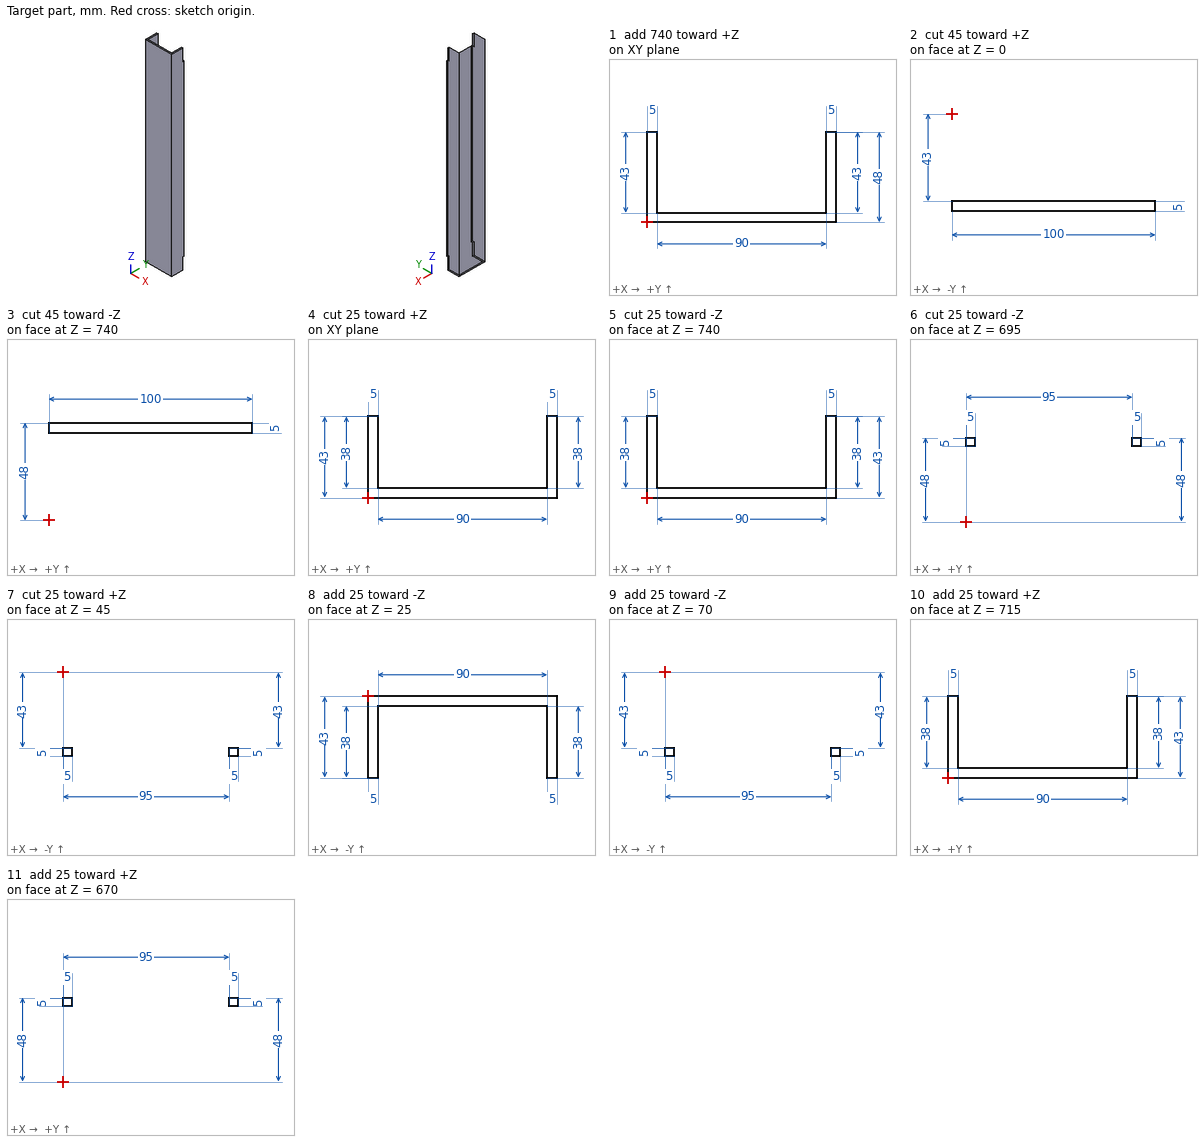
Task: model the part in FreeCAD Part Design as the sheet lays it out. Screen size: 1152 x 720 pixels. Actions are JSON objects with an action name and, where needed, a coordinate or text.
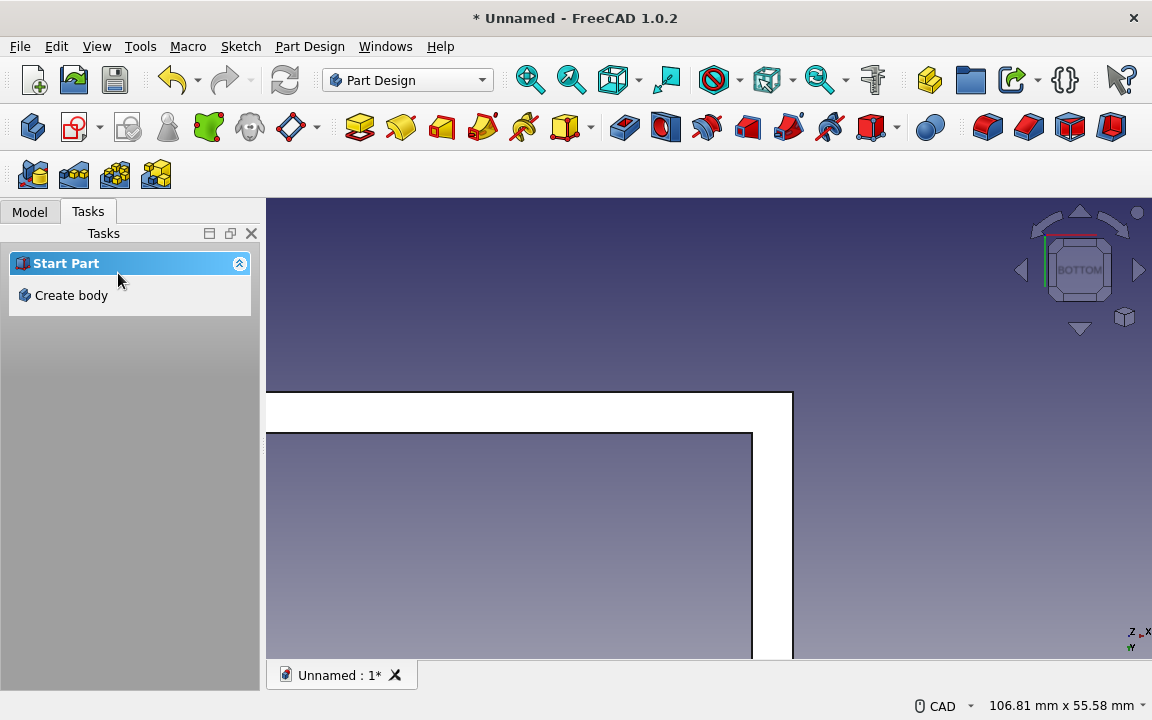
{"action": "left_click", "coordinate": [531, 80]}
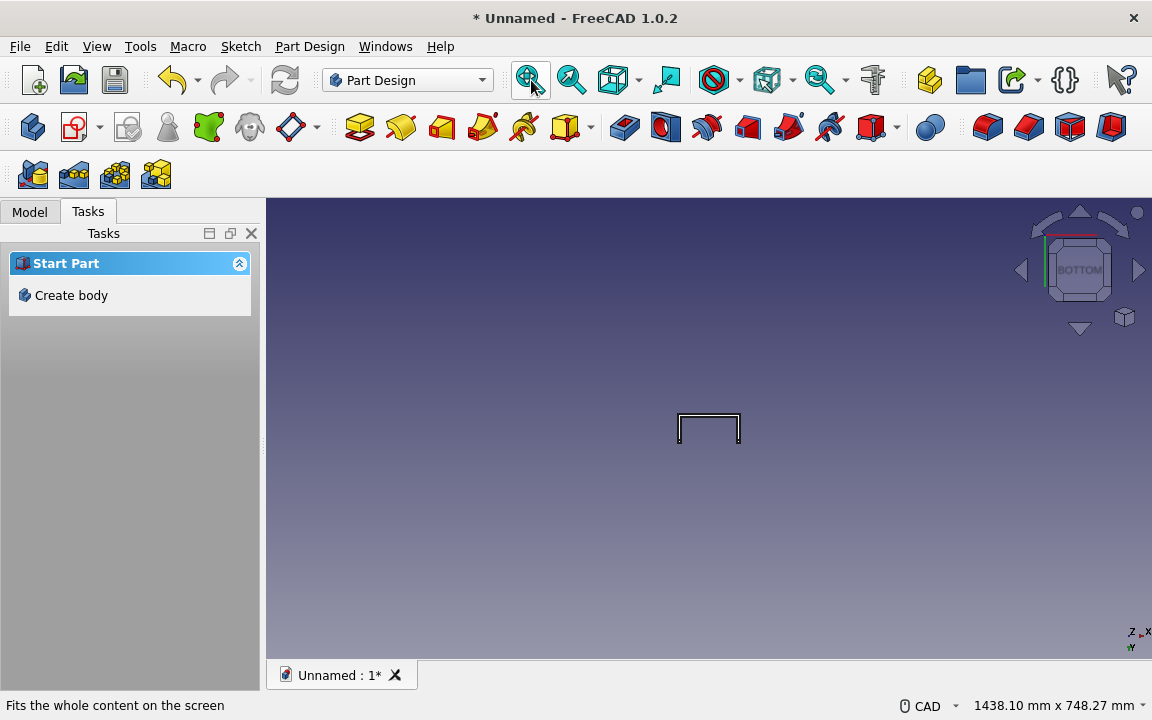
{"action": "key", "text": "0"}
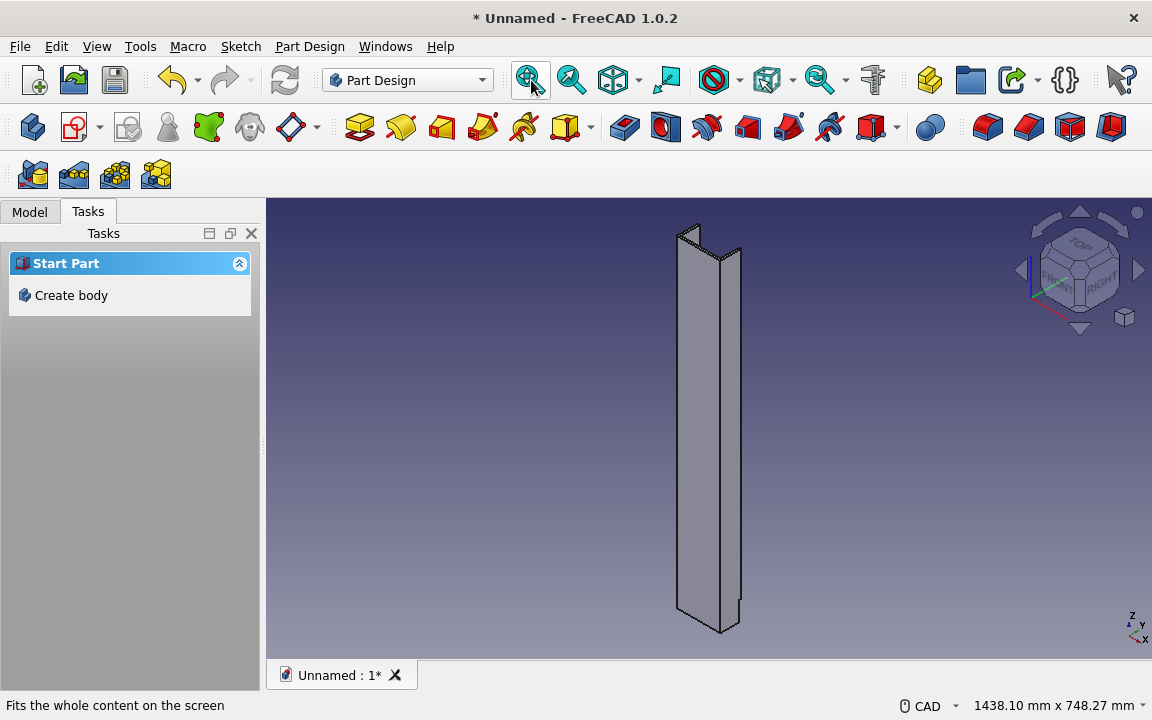
{"action": "scroll", "coordinate": [719, 257], "scroll_direction": "up", "scroll_amount": 13}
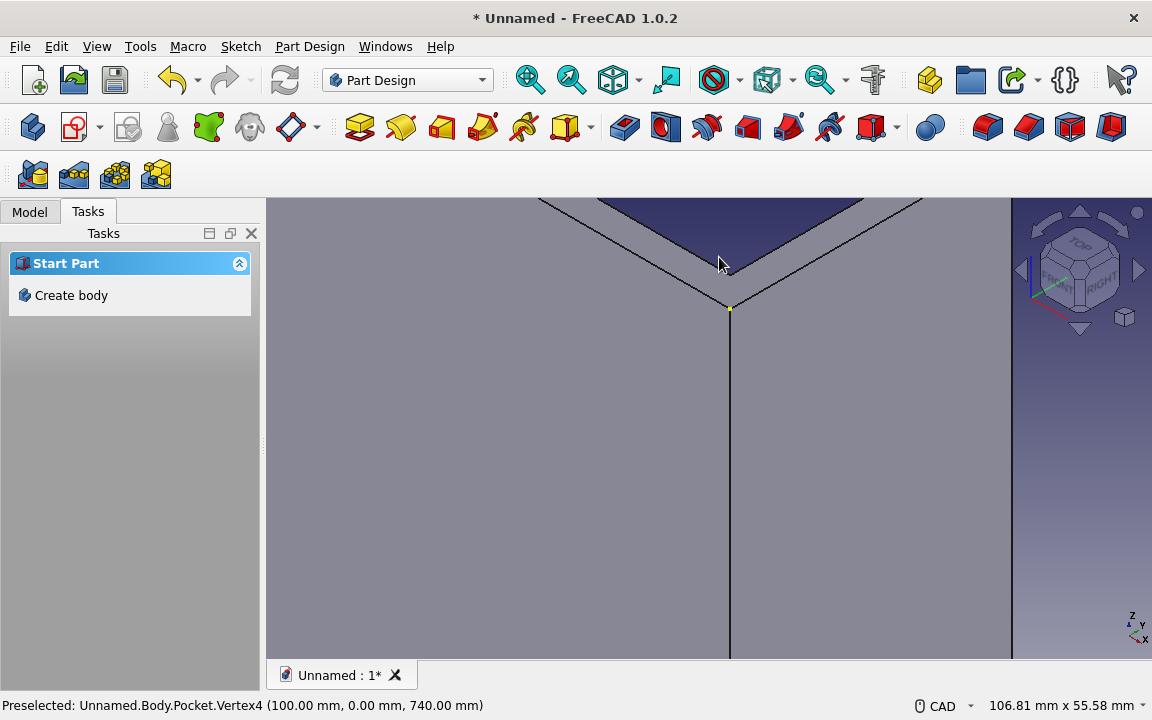
{"action": "left_click", "coordinate": [709, 272]}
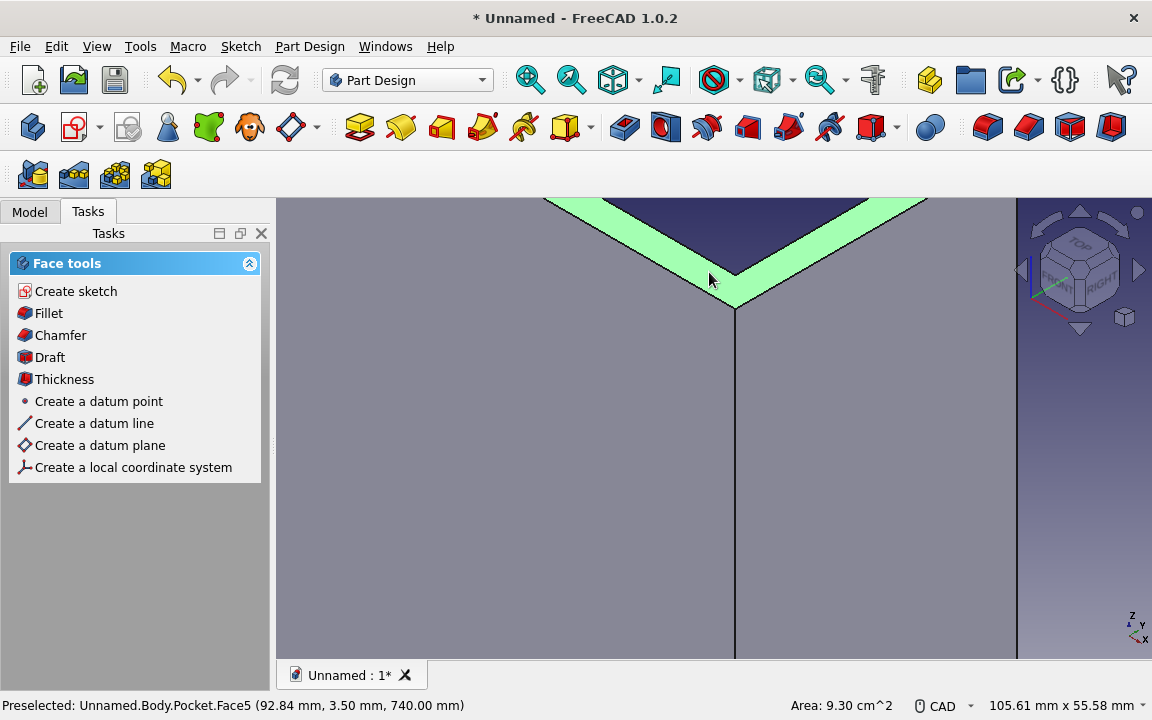
{"action": "left_click", "coordinate": [74, 128]}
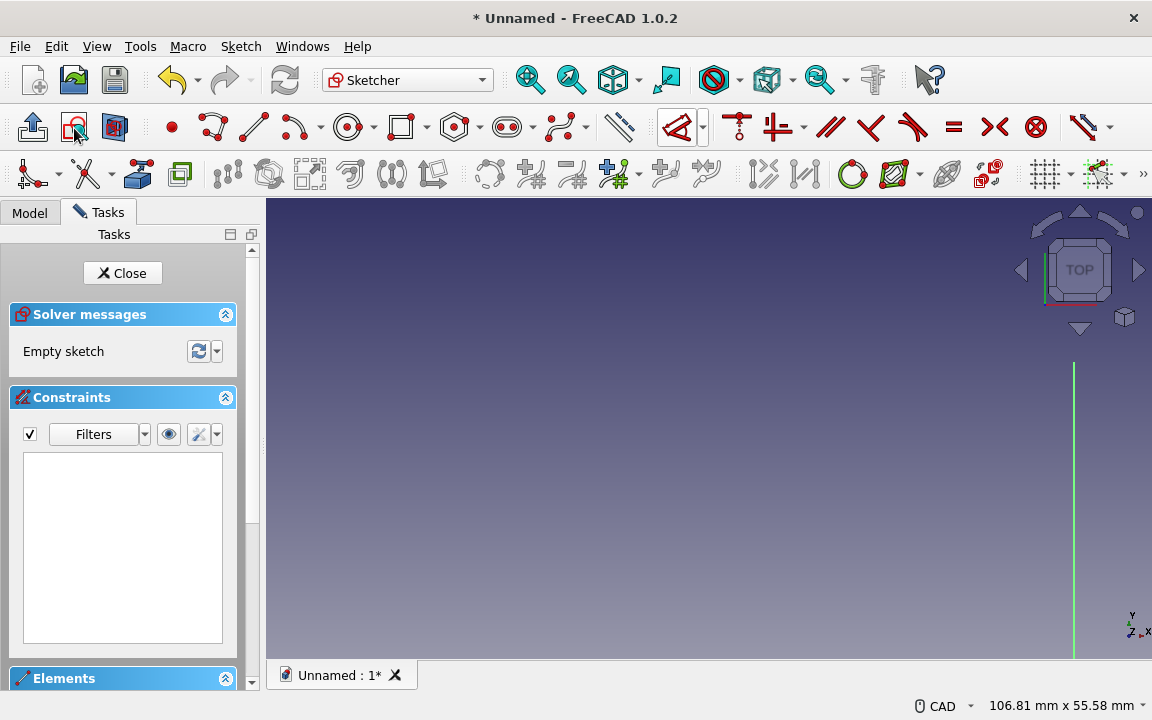
{"action": "scroll", "coordinate": [640, 428], "scroll_direction": "down", "scroll_amount": 5}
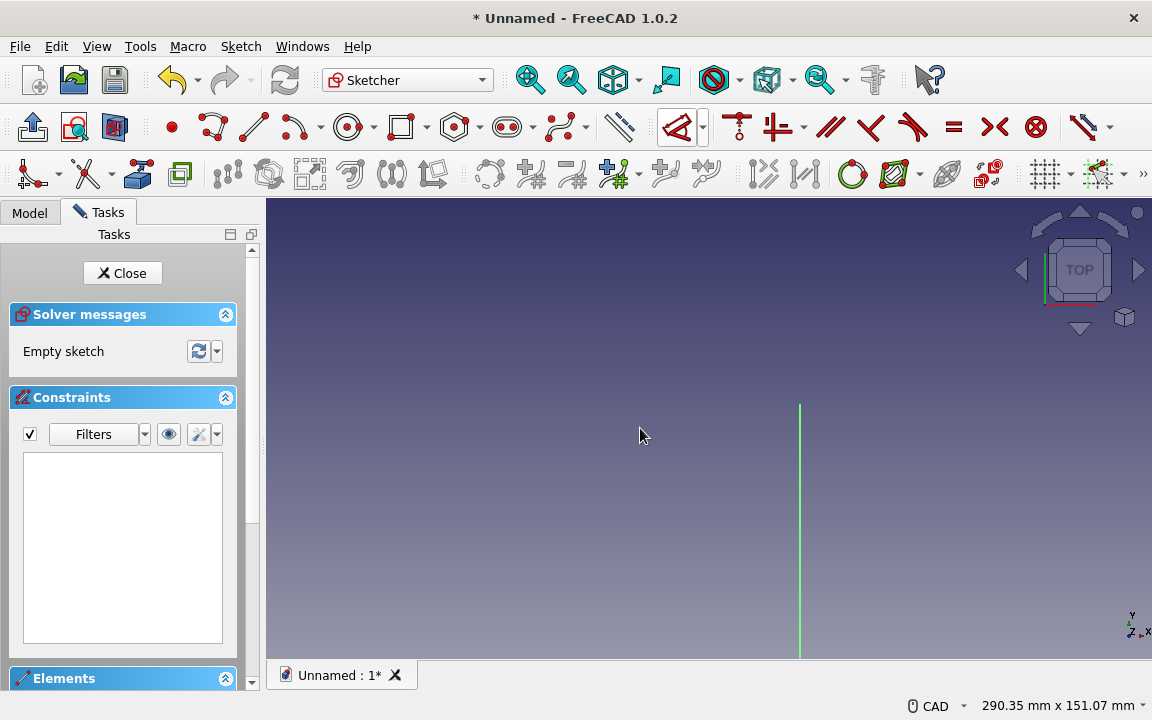
{"action": "scroll", "coordinate": [640, 428], "scroll_direction": "down", "scroll_amount": 5}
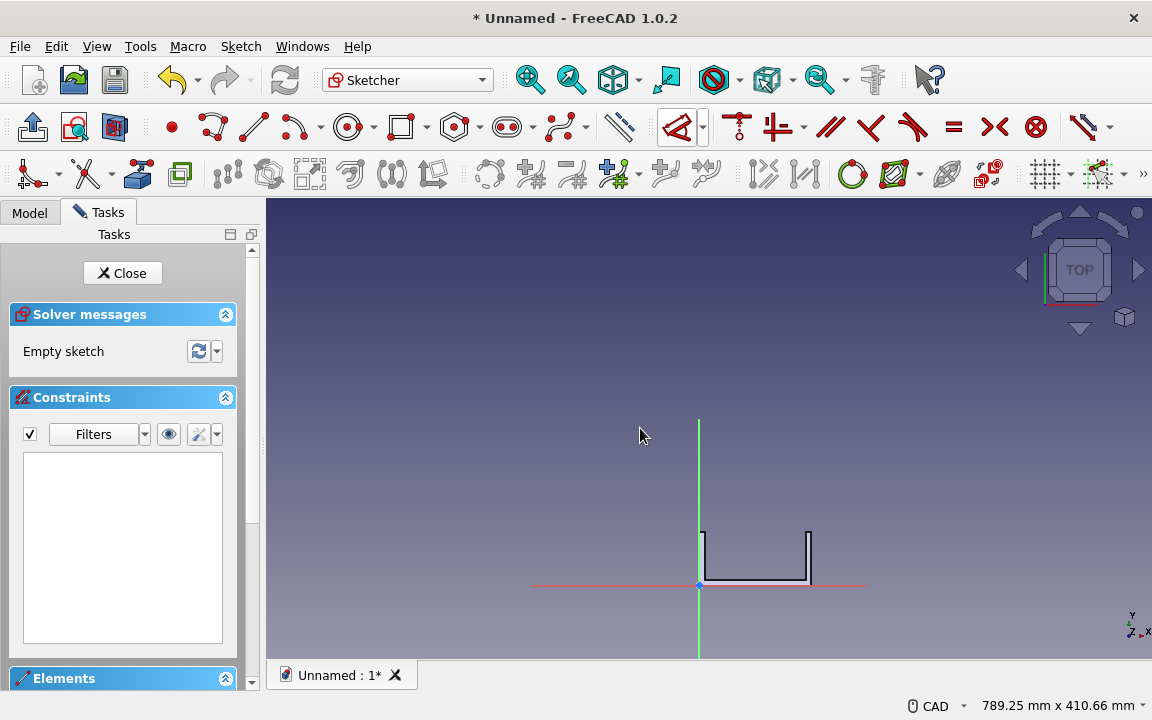
{"action": "scroll", "coordinate": [793, 602], "scroll_direction": "up", "scroll_amount": 7}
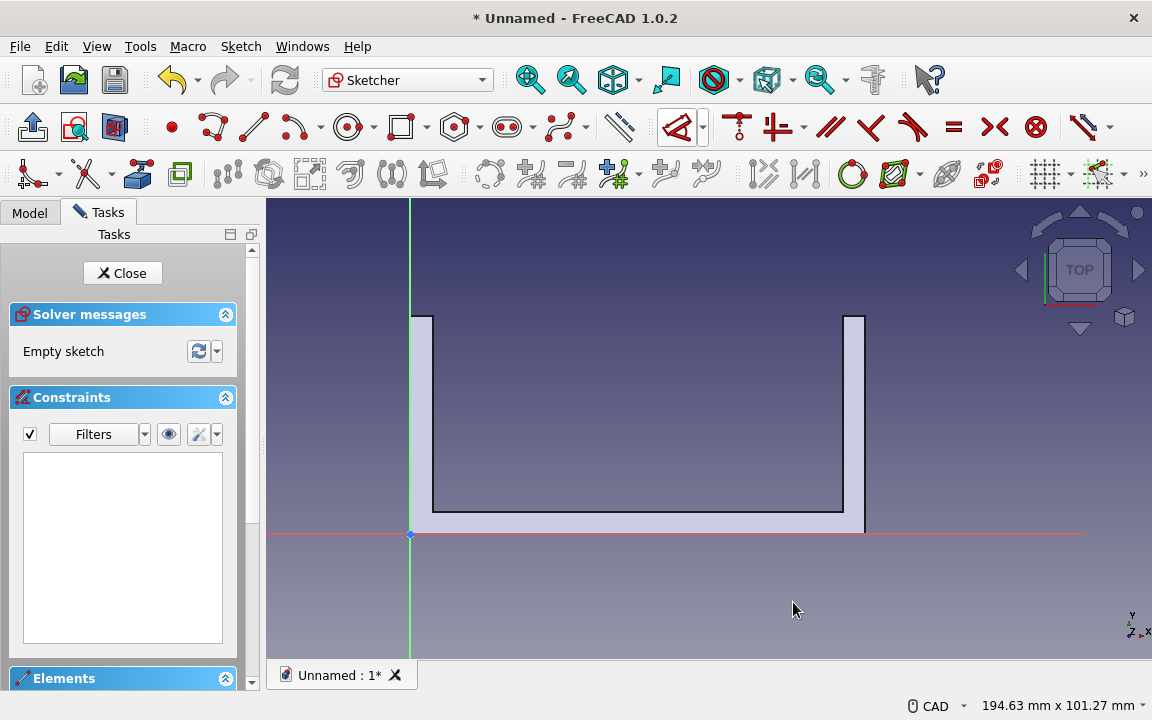
{"action": "left_click", "coordinate": [400, 128]}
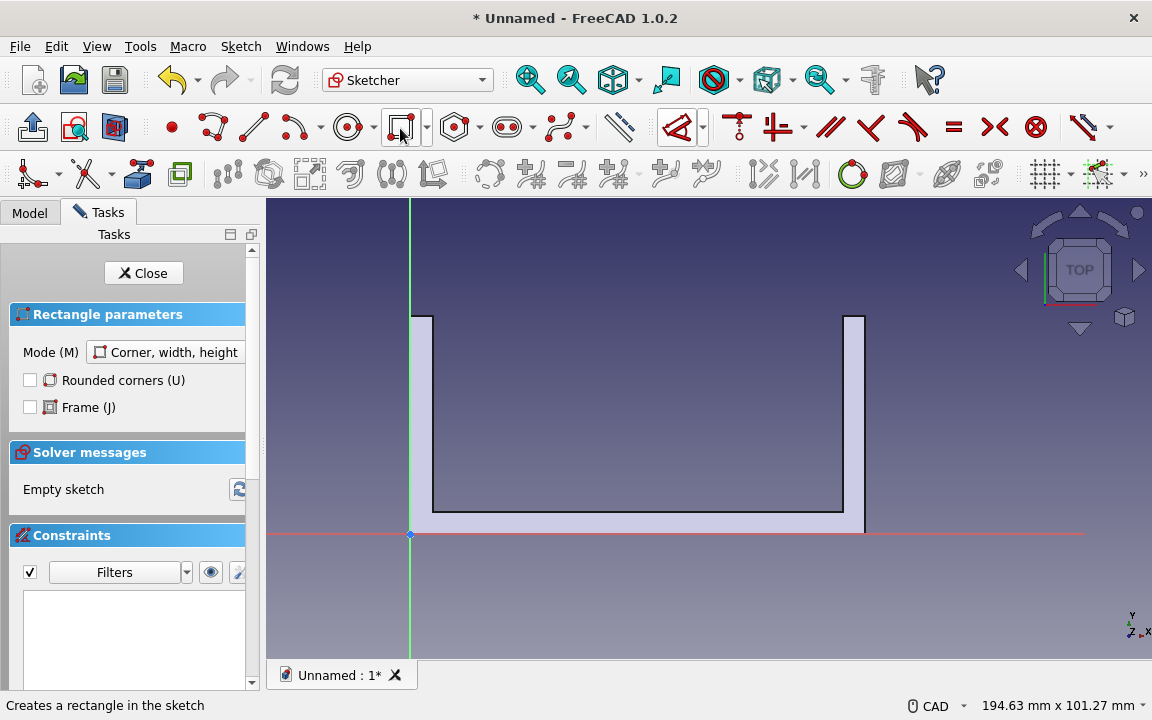
{"action": "left_click", "coordinate": [410, 316]}
{"action": "mouse_move", "coordinate": [865, 339]}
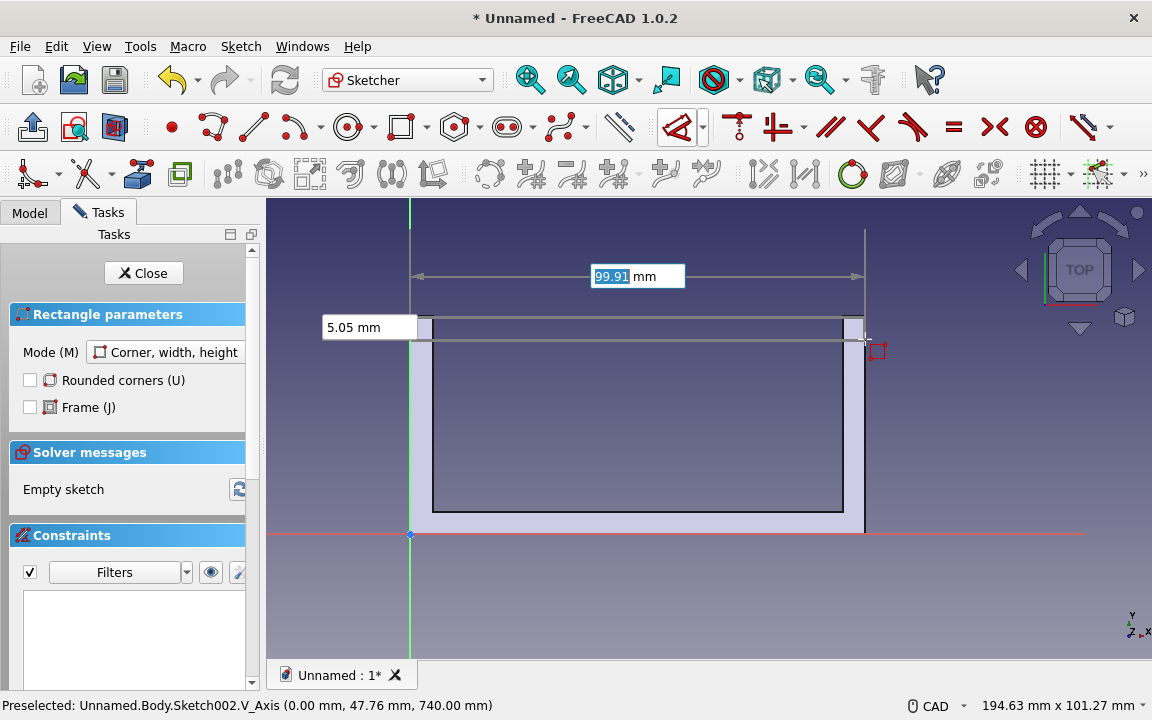
{"action": "type", "text": "100"}
{"action": "key", "text": "Tab"}
{"action": "type", "text": "5"}
{"action": "key", "text": "Return"}
{"action": "key", "text": "Escape"}